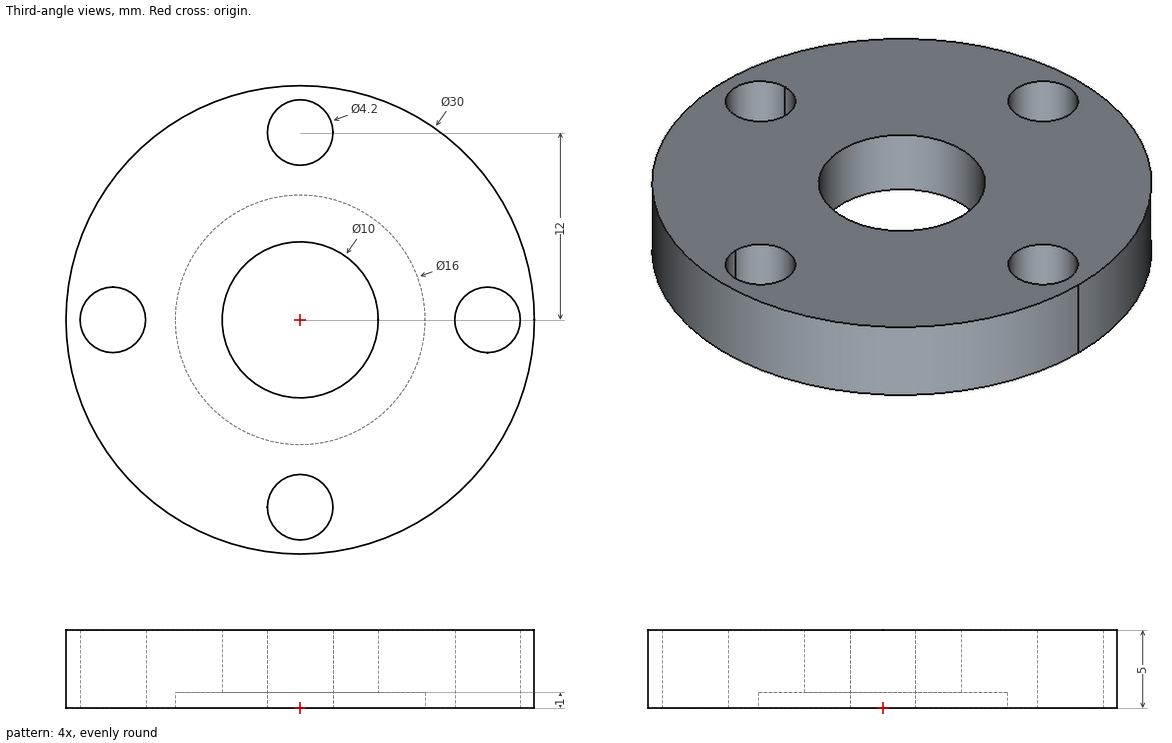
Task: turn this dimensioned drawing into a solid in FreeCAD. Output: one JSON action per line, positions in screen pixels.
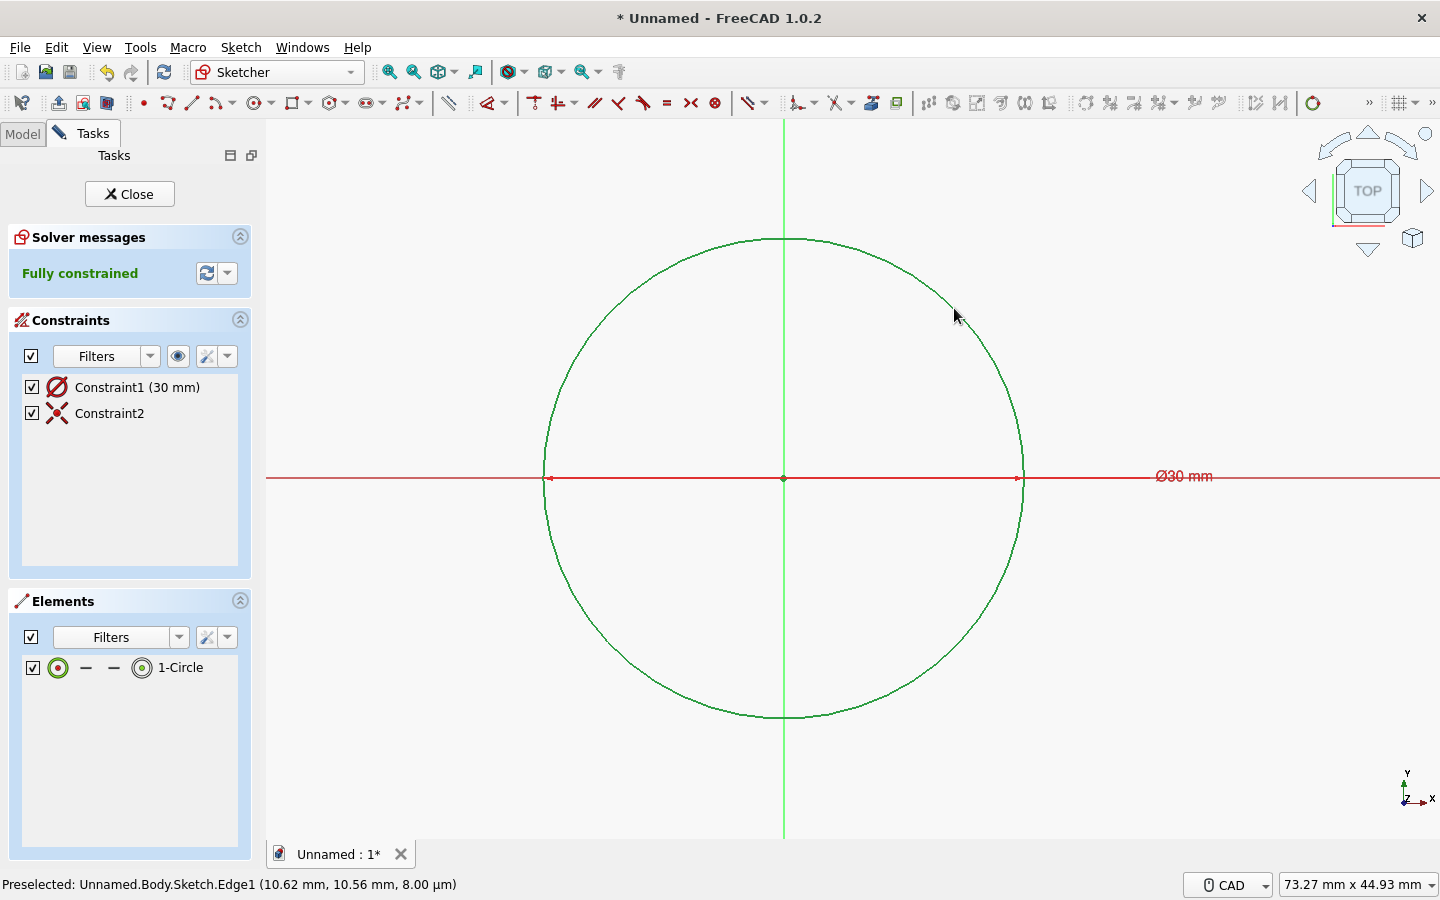
{"action": "left_click", "coordinate": [130, 194]}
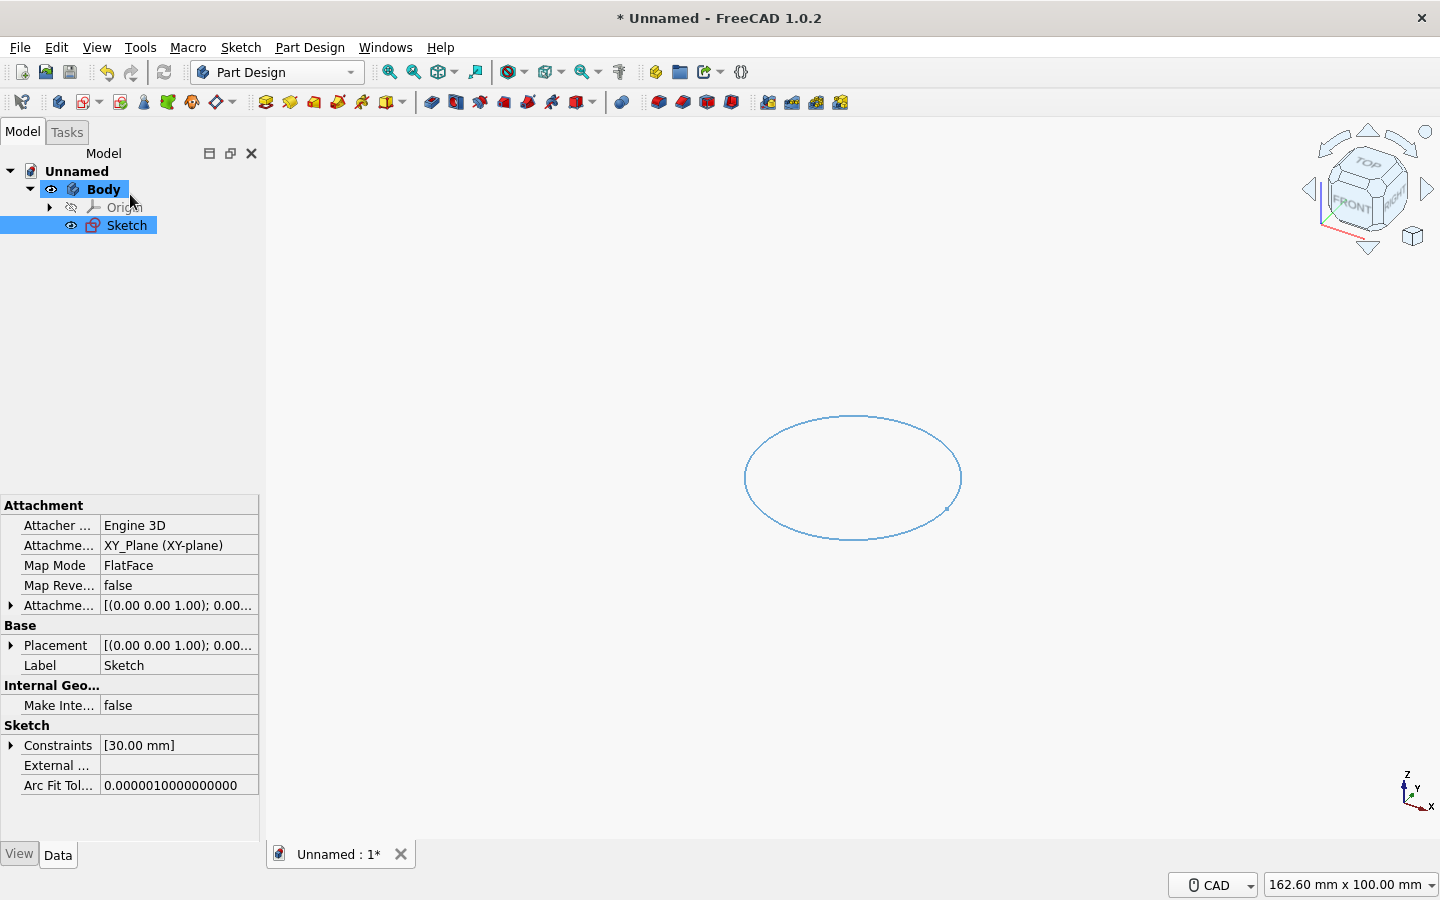
{"action": "left_click", "coordinate": [266, 102]}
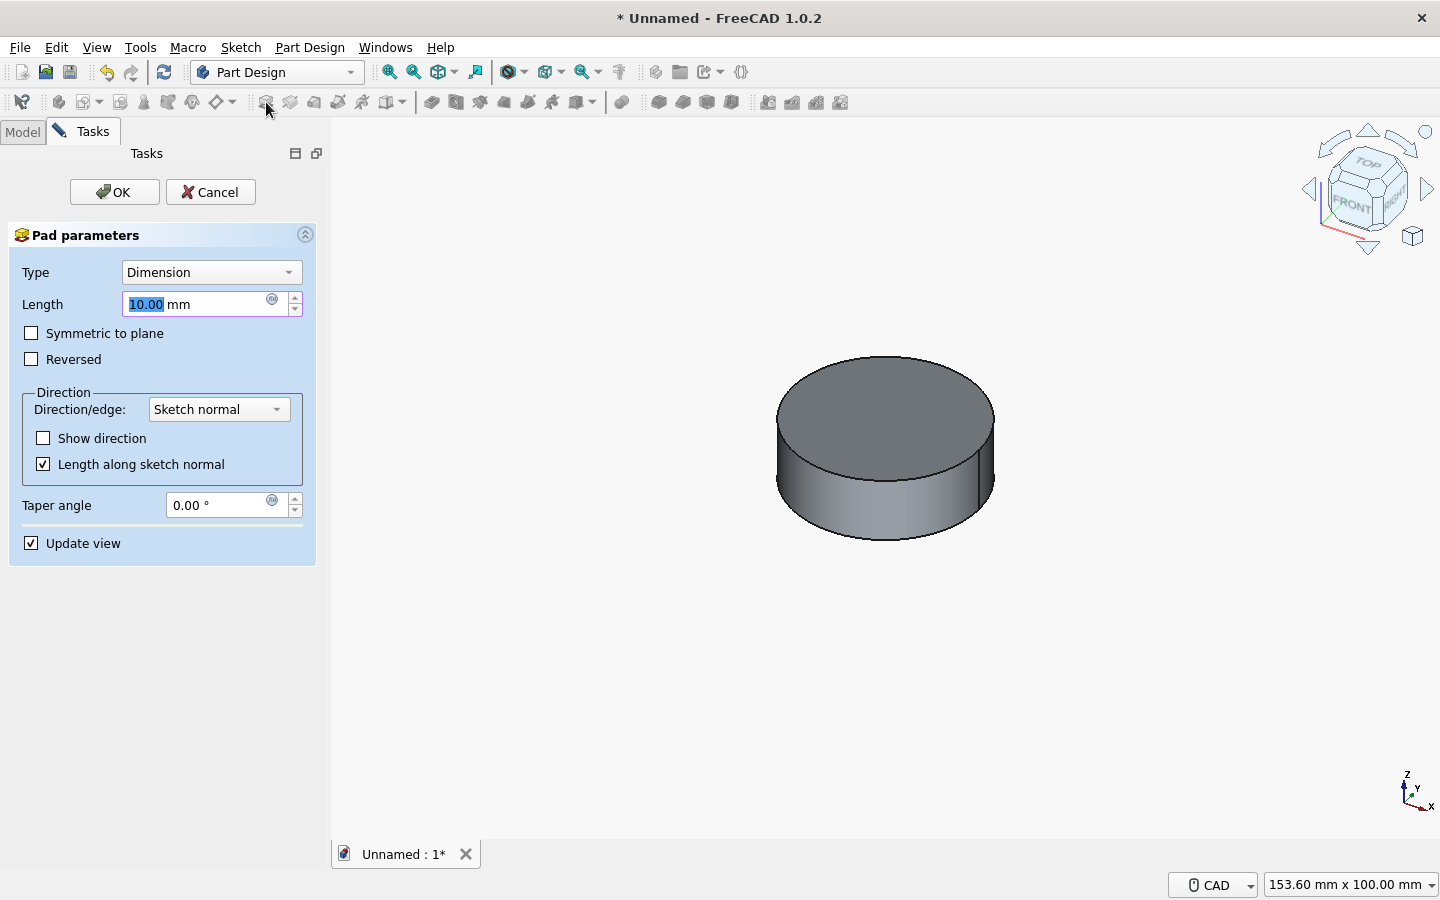
{"action": "type", "text": "5"}
{"action": "key", "text": "Tab"}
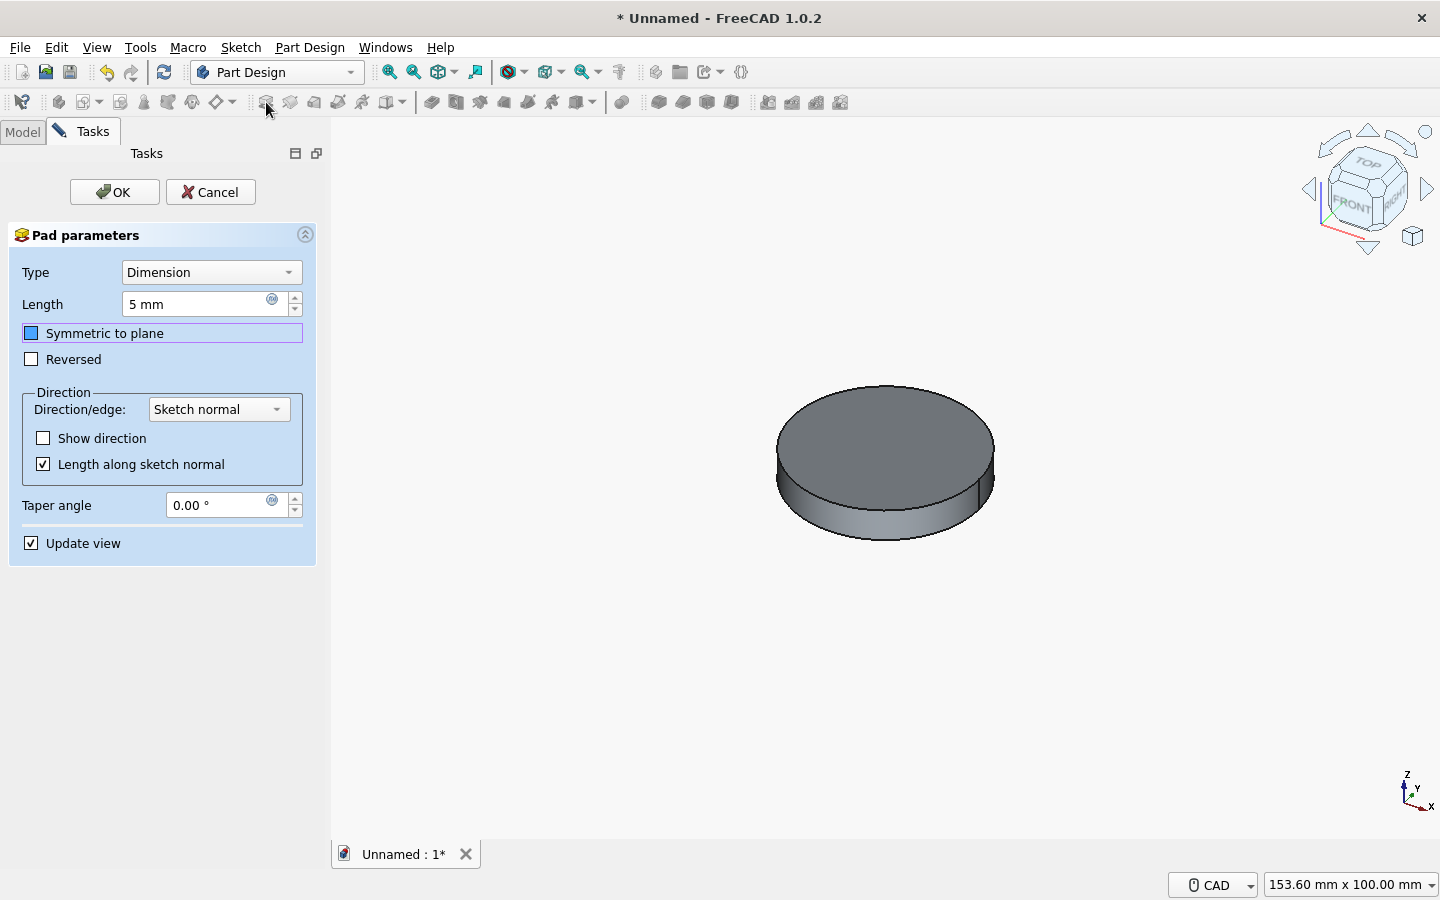
{"action": "left_click", "coordinate": [115, 192]}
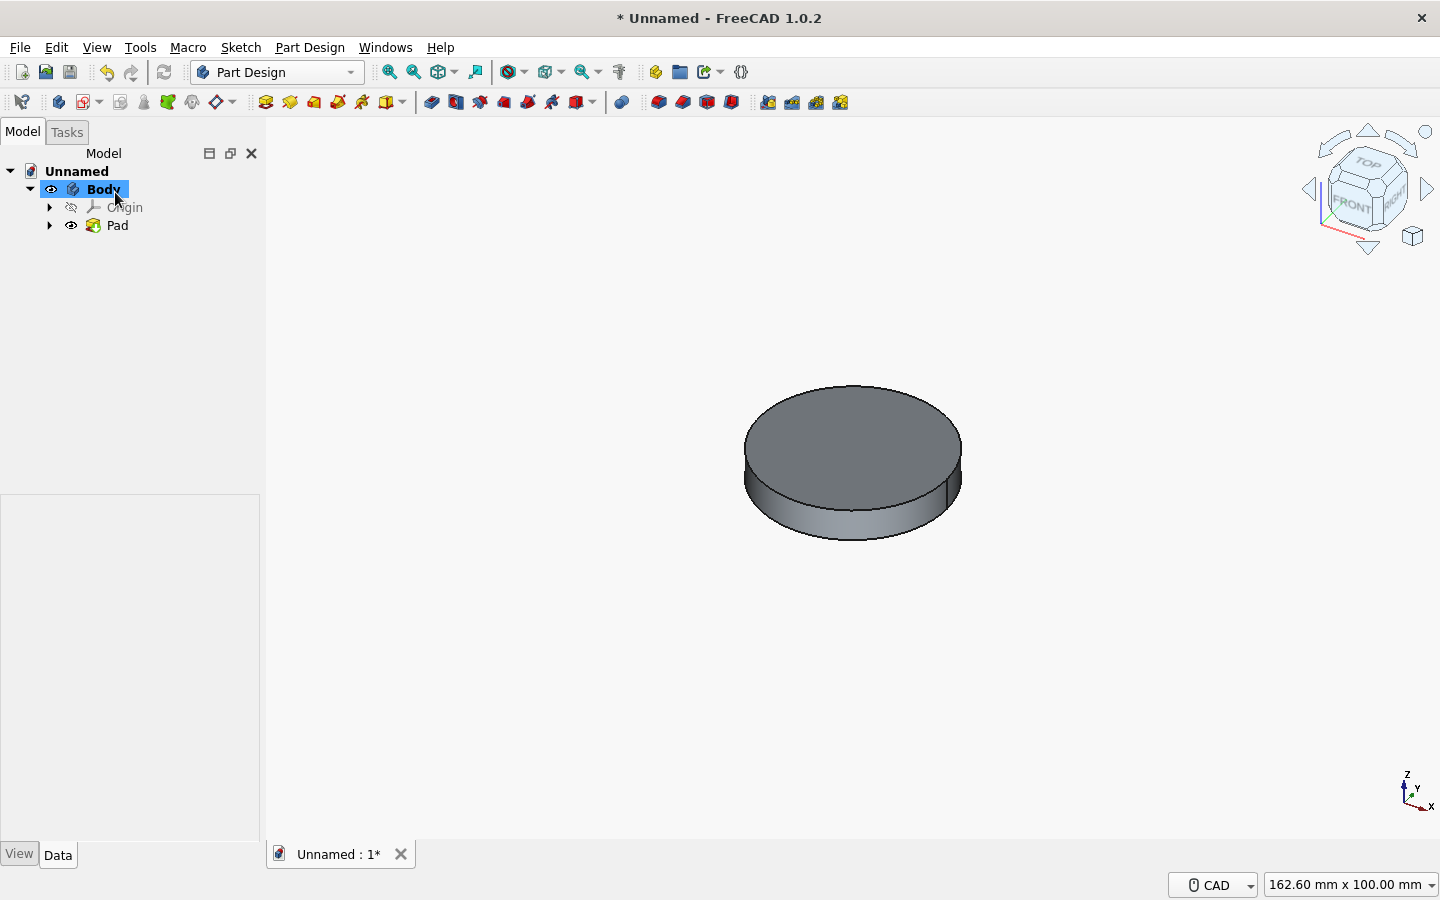
{"action": "left_click", "coordinate": [390, 72]}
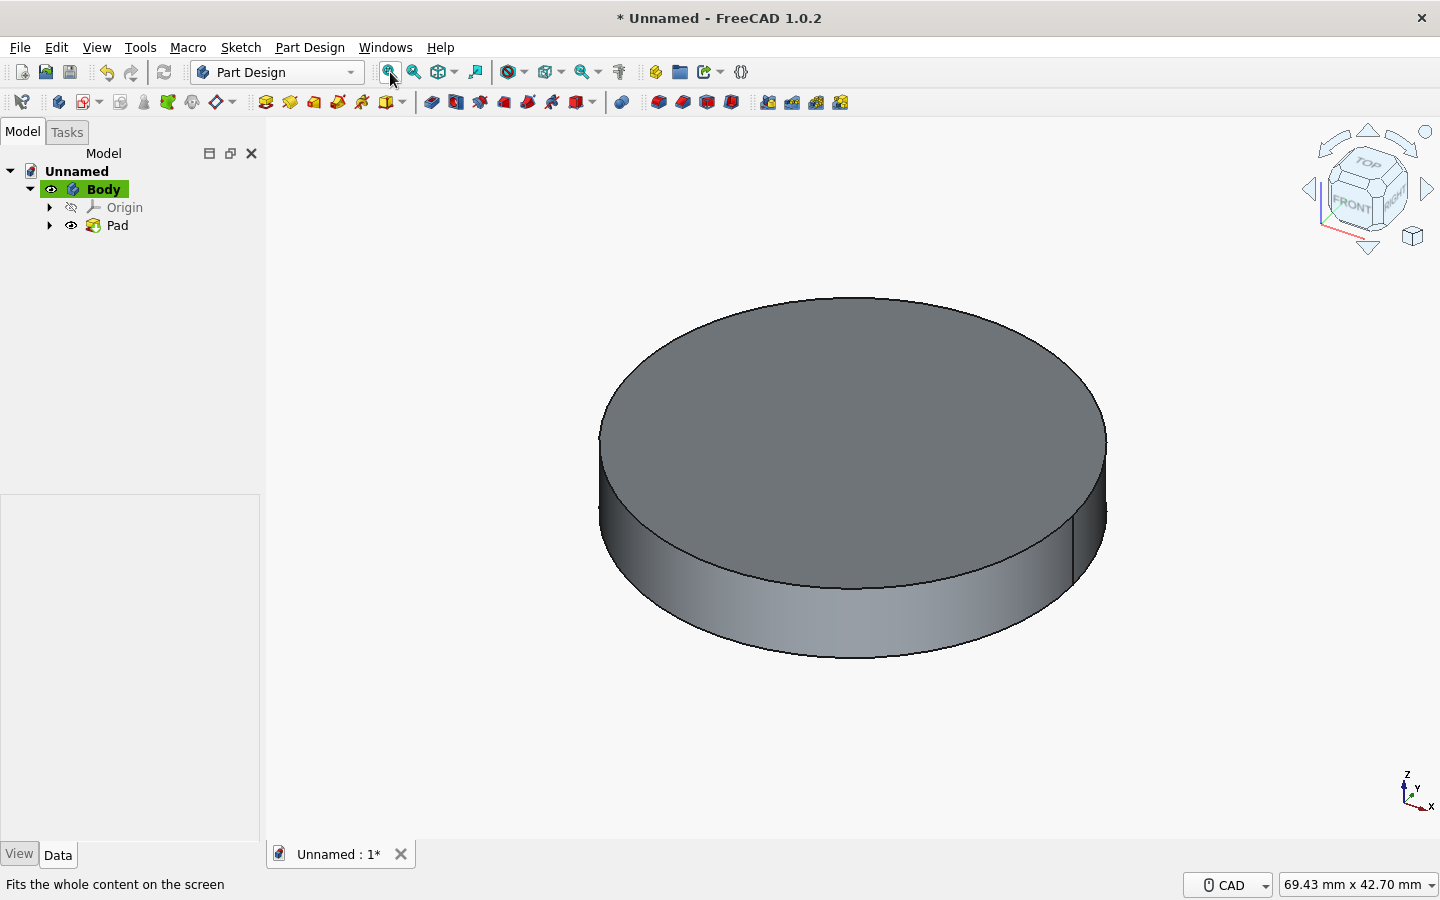
{"action": "left_click", "coordinate": [853, 442]}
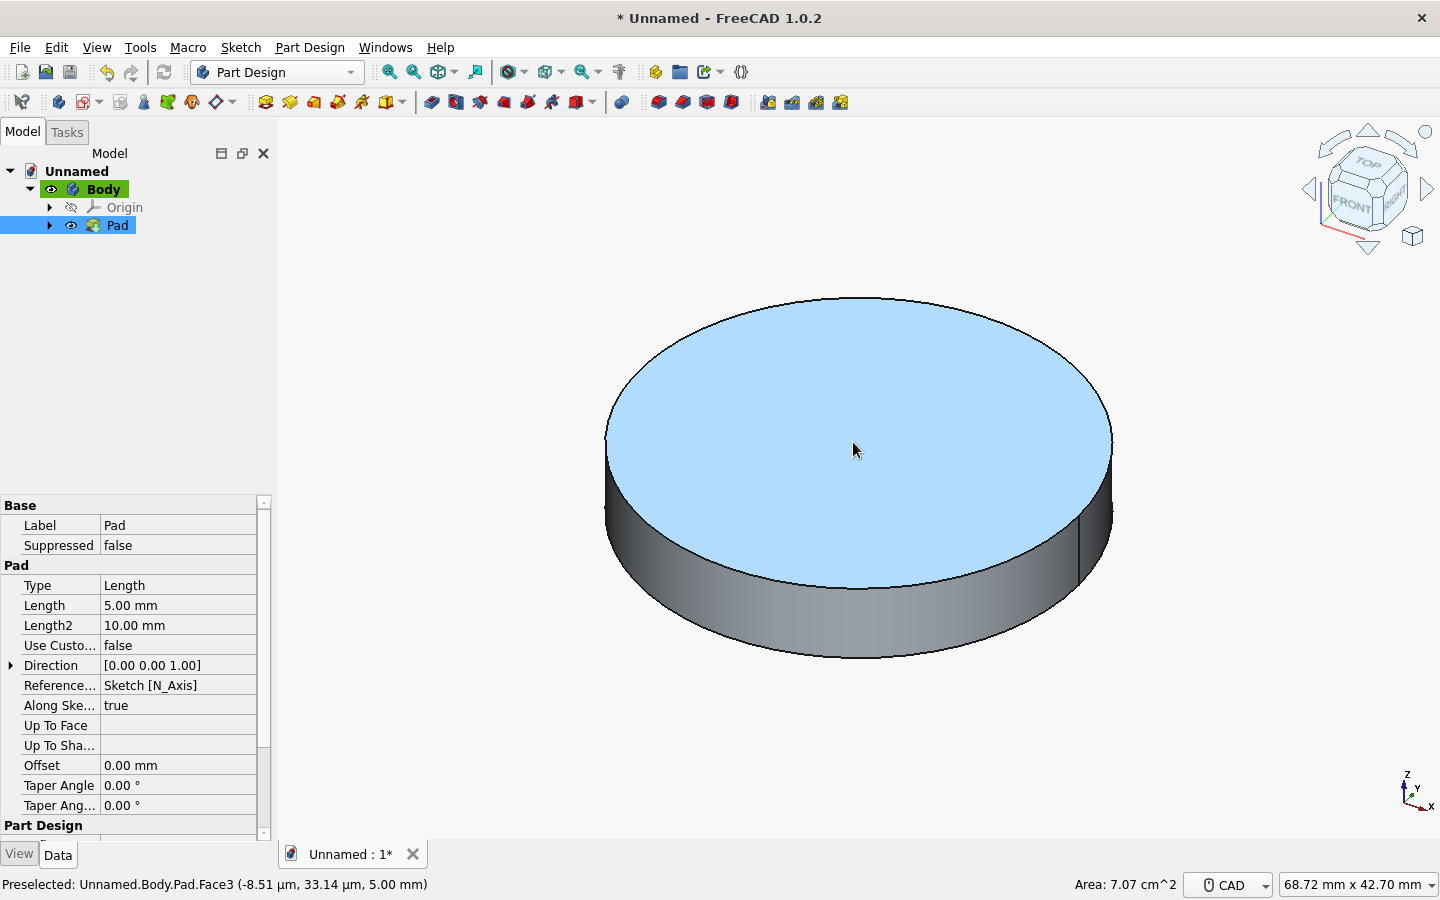
{"action": "left_click", "coordinate": [84, 102]}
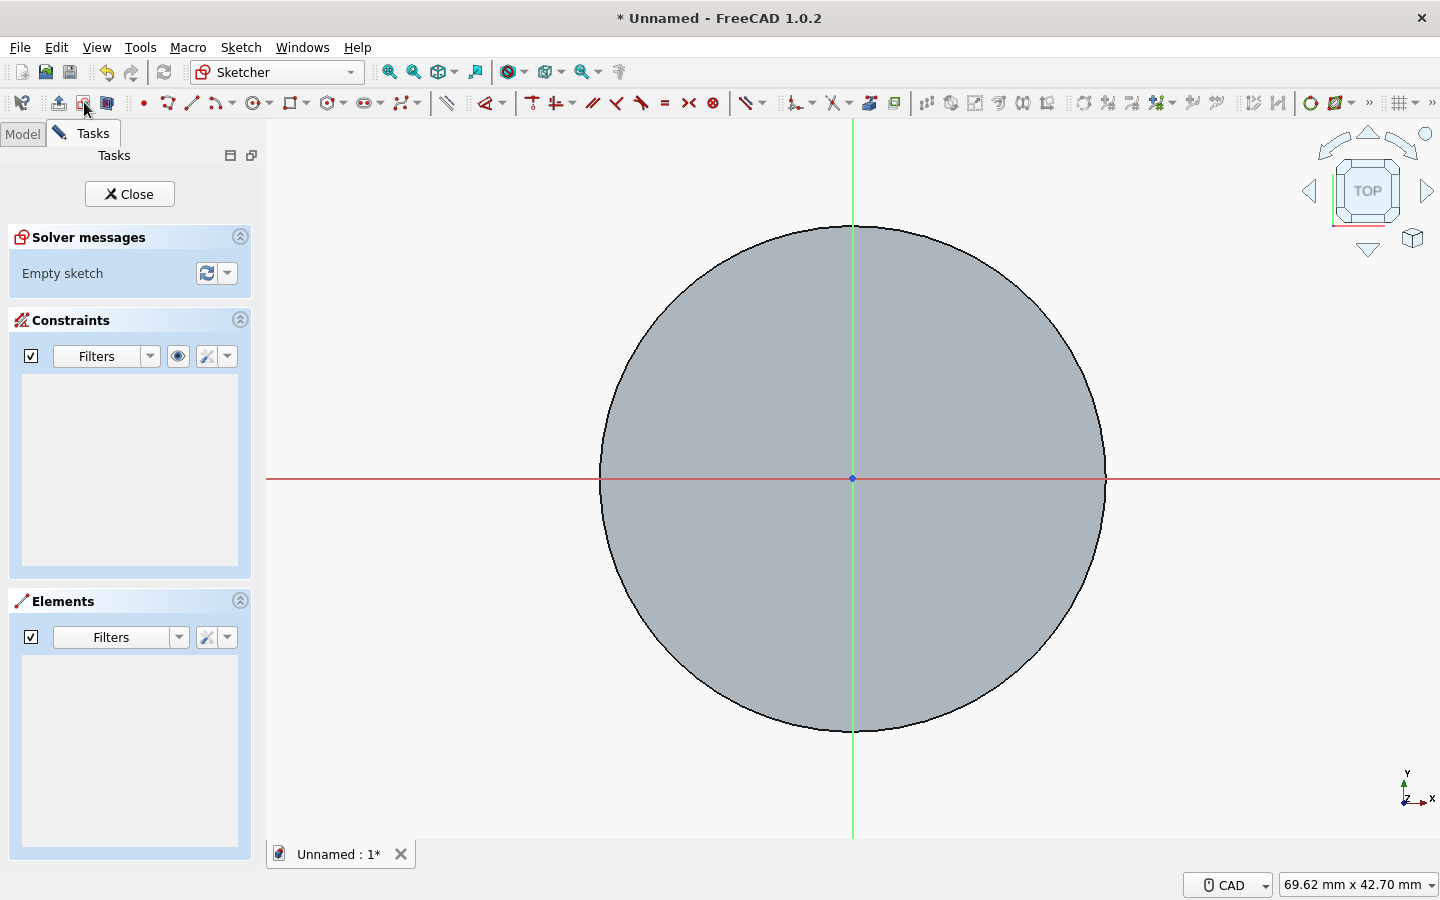
{"action": "scroll", "coordinate": [866, 237], "scroll_direction": "up", "scroll_amount": 9}